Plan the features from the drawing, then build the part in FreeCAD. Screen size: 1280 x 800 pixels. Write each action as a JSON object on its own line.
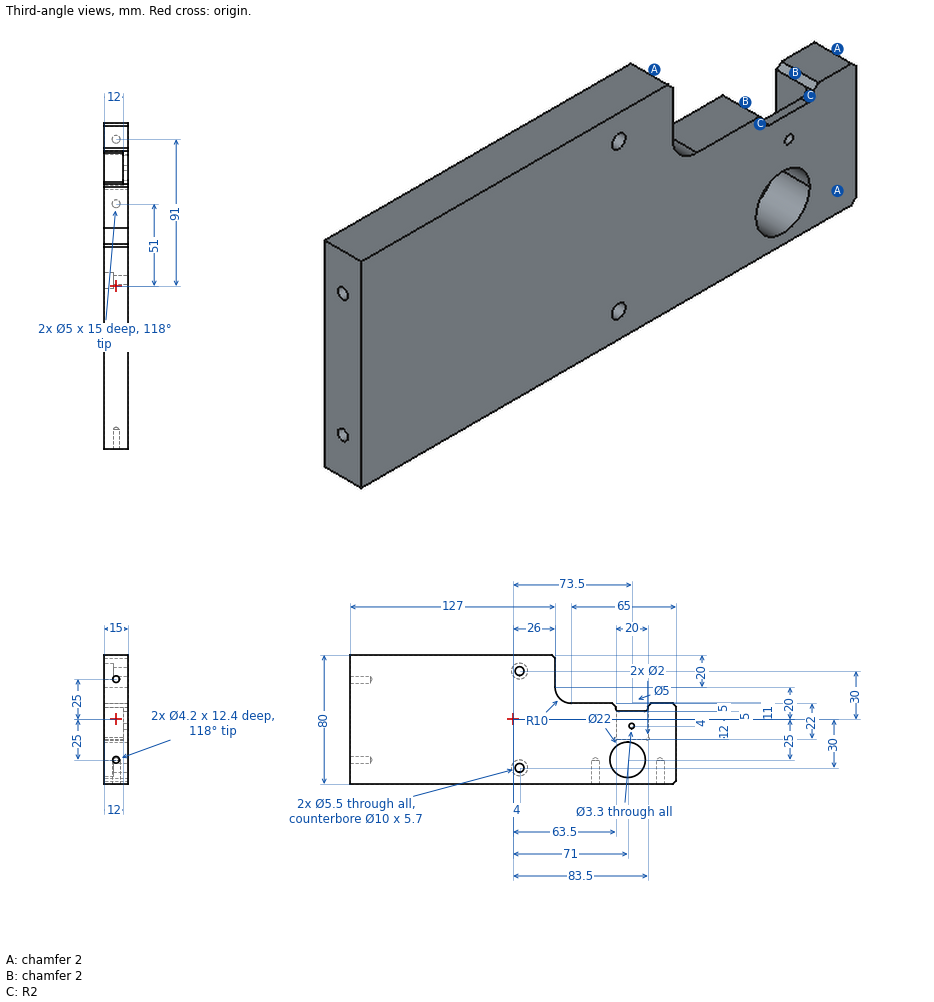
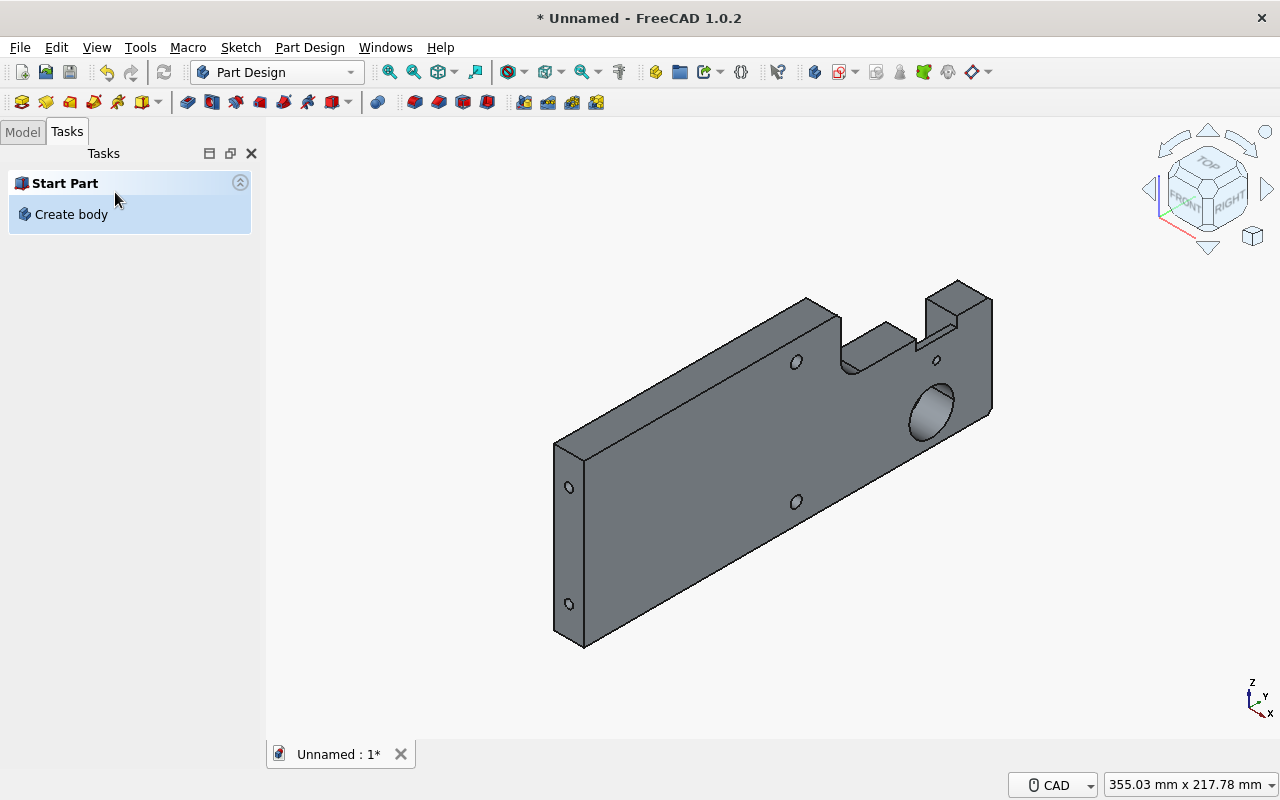
{"action": "left_click", "coordinate": [942, 306]}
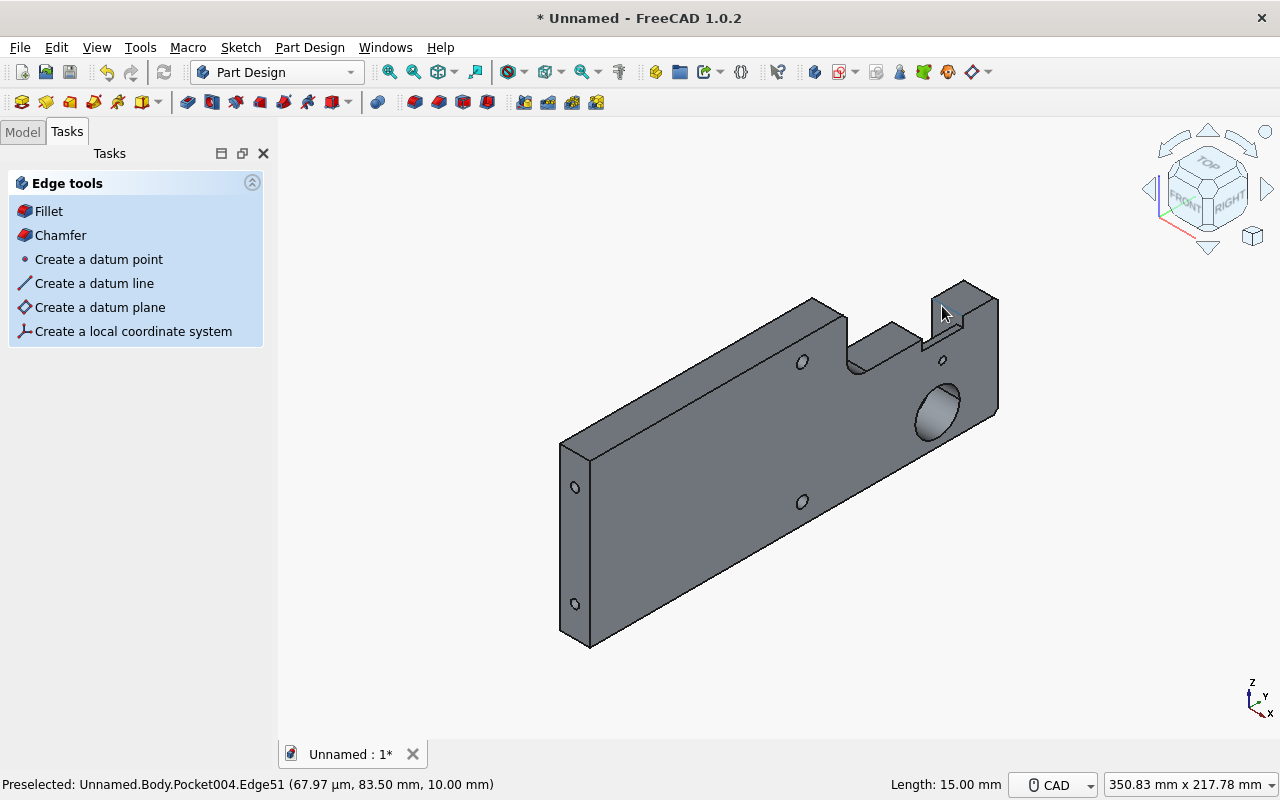
{"action": "key", "text": "2"}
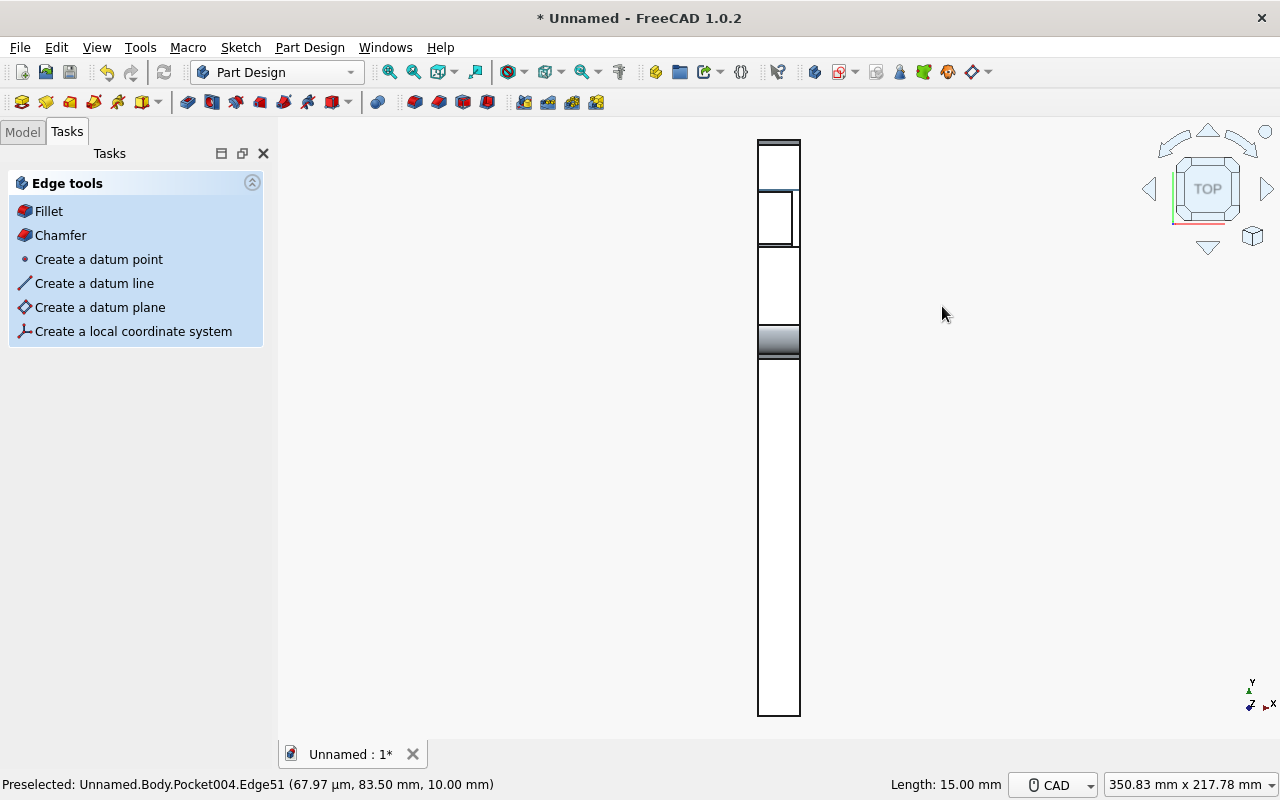
{"action": "left_click", "coordinate": [779, 246], "text": "ctrl"}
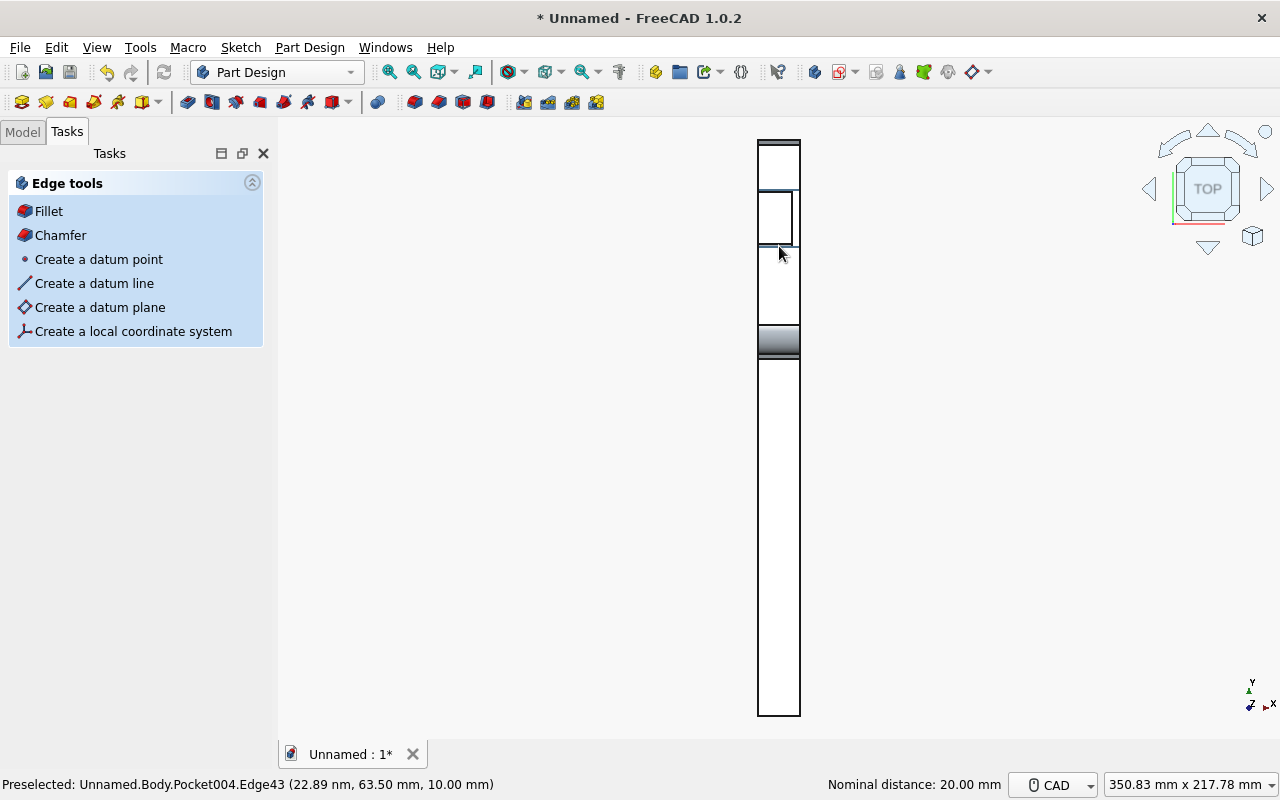
{"action": "left_click", "coordinate": [440, 102]}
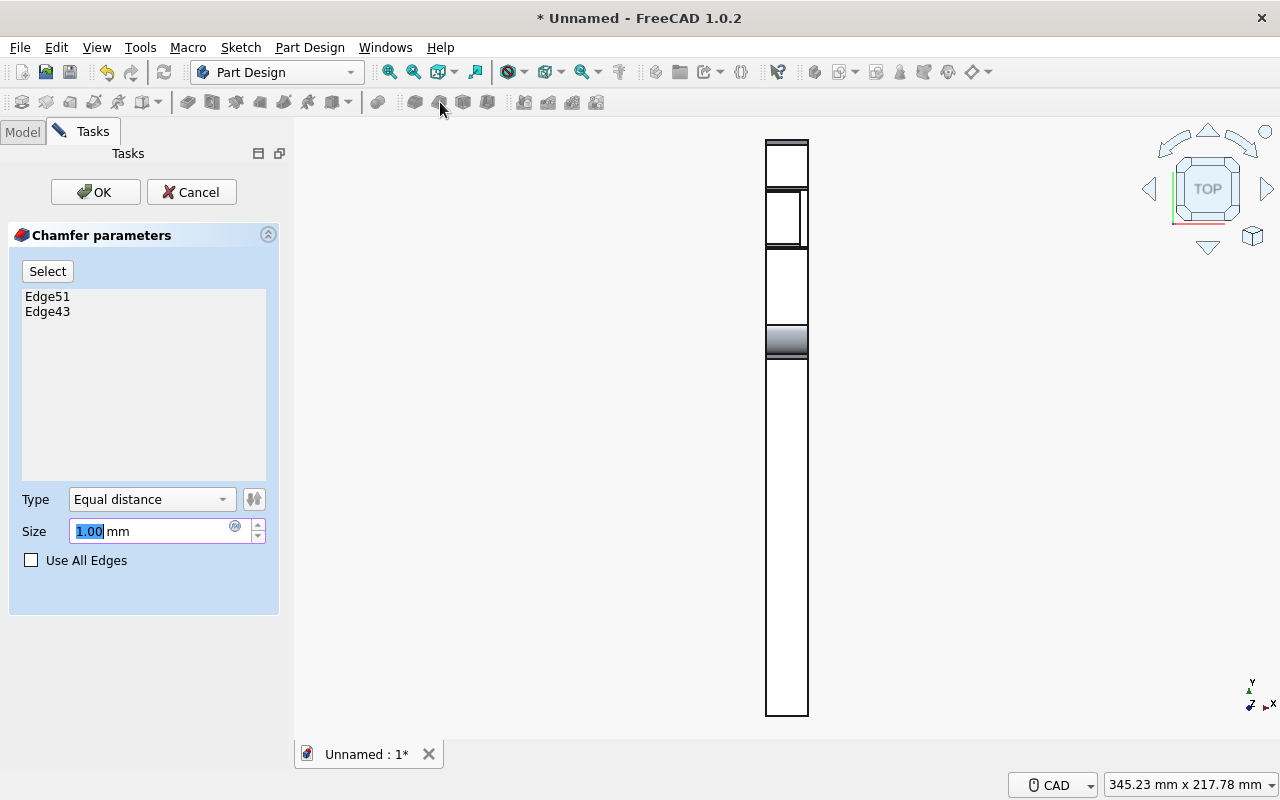
{"action": "type", "text": "2"}
{"action": "key", "text": "Tab"}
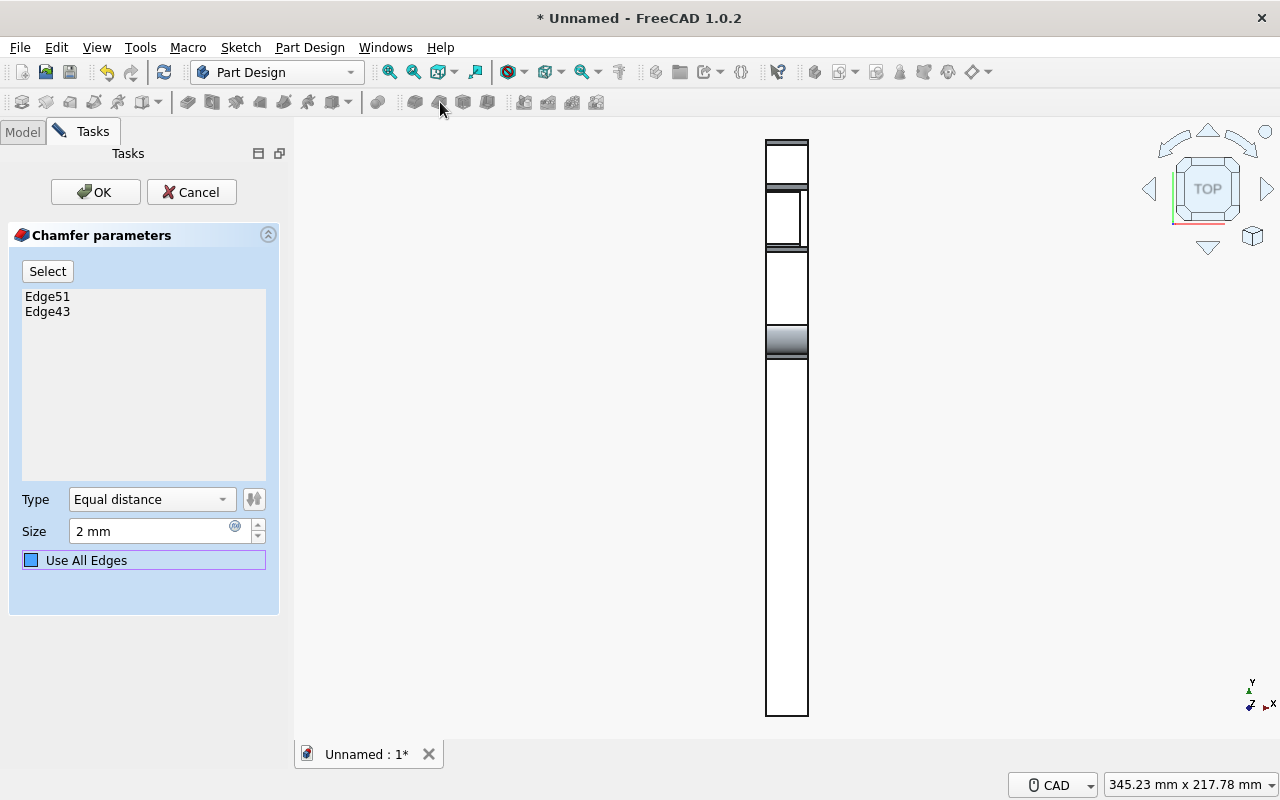
{"action": "left_click", "coordinate": [96, 192]}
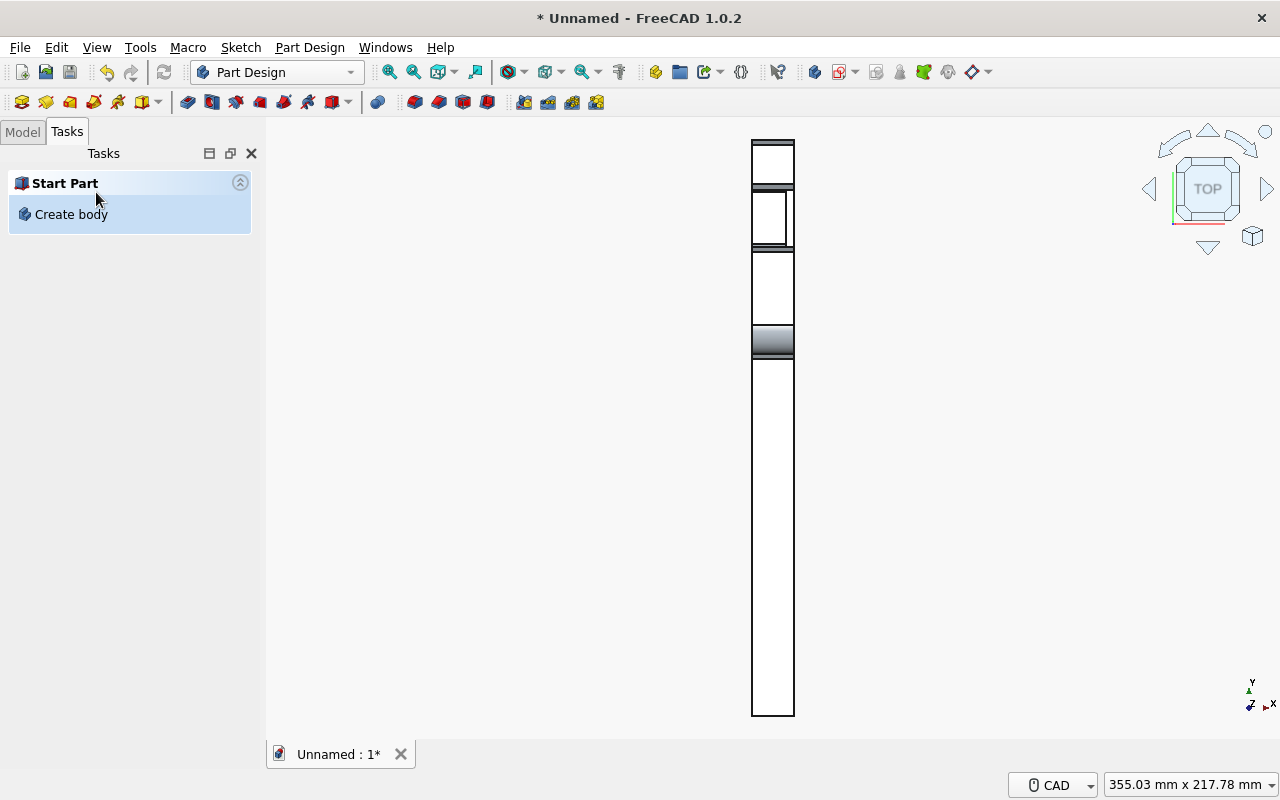
{"action": "scroll", "coordinate": [790, 246], "scroll_direction": "up", "scroll_amount": 8}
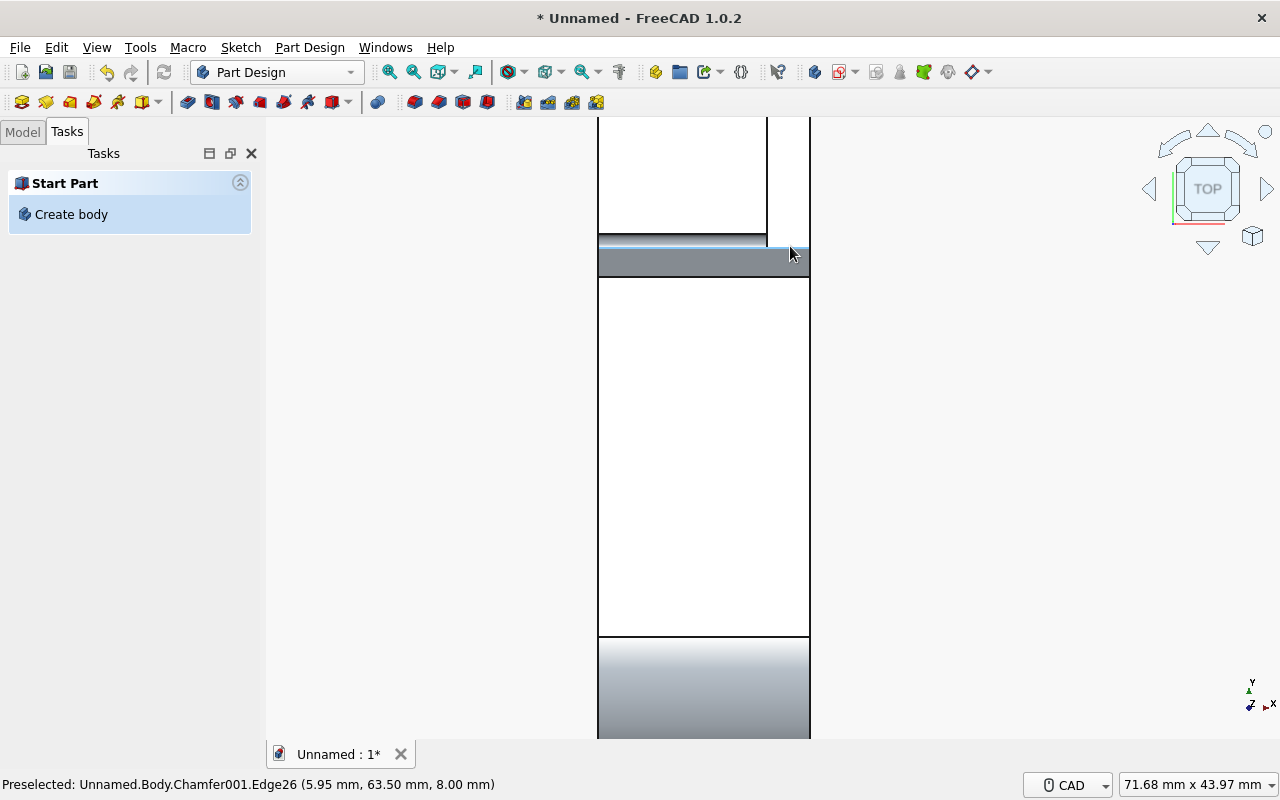
{"action": "left_click", "coordinate": [390, 72]}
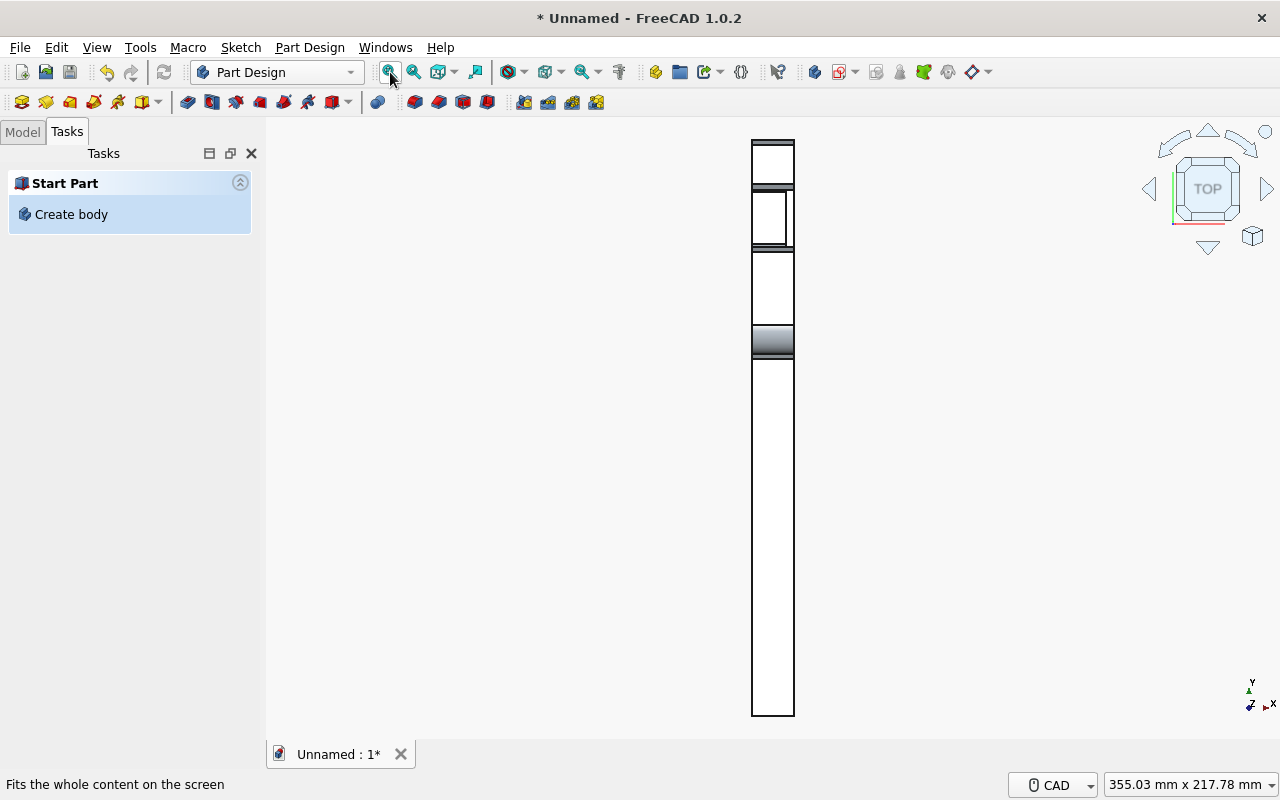
{"action": "key", "text": "0"}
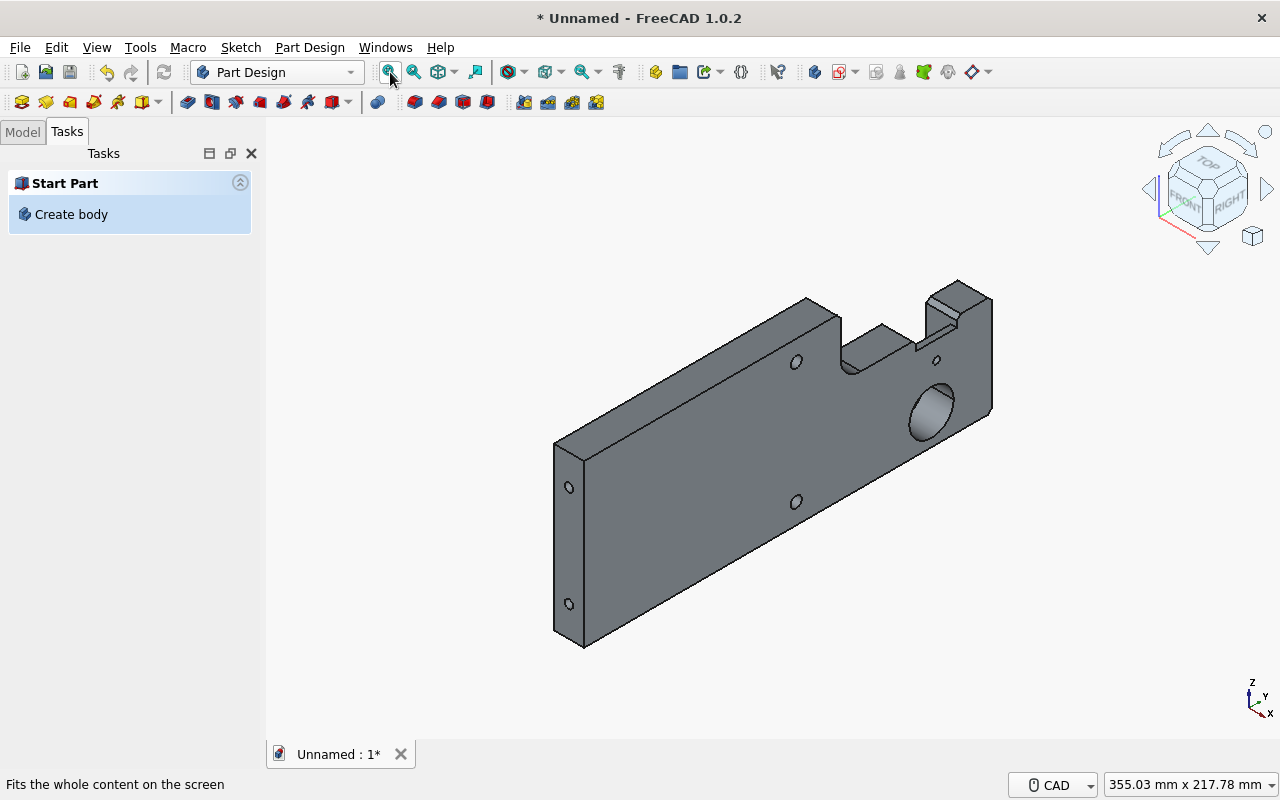
{"action": "scroll", "coordinate": [913, 348], "scroll_direction": "up", "scroll_amount": 8}